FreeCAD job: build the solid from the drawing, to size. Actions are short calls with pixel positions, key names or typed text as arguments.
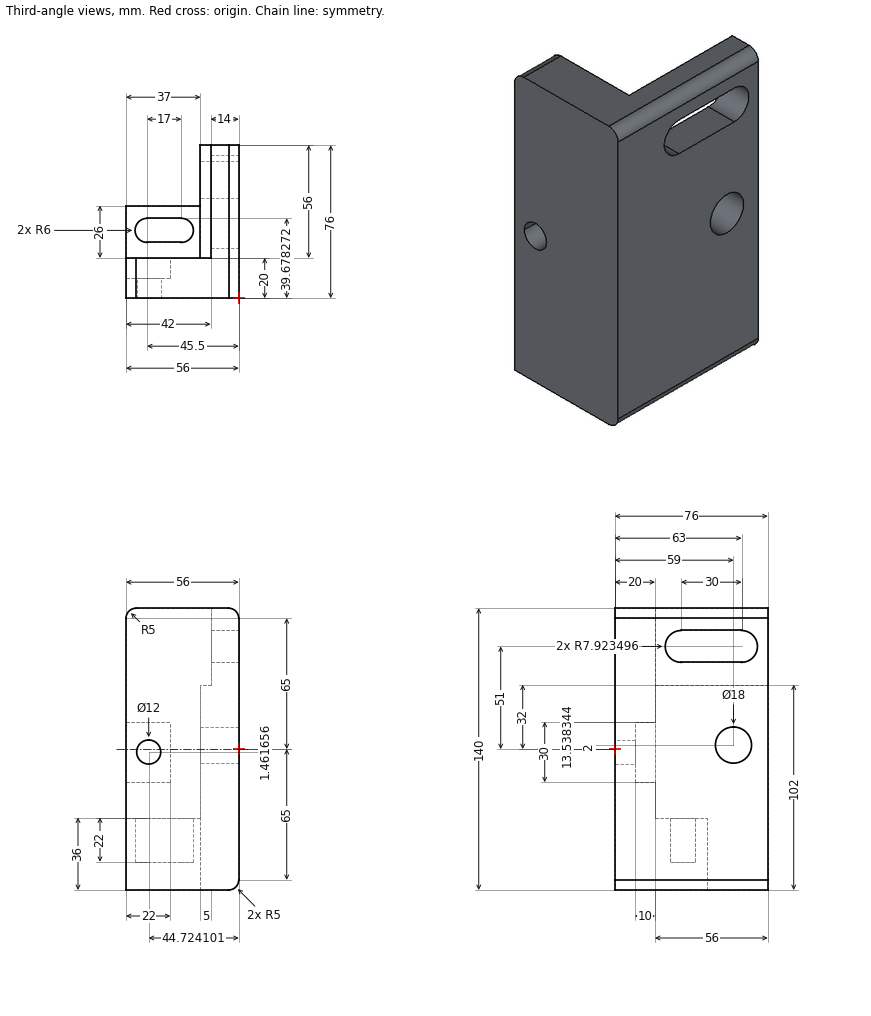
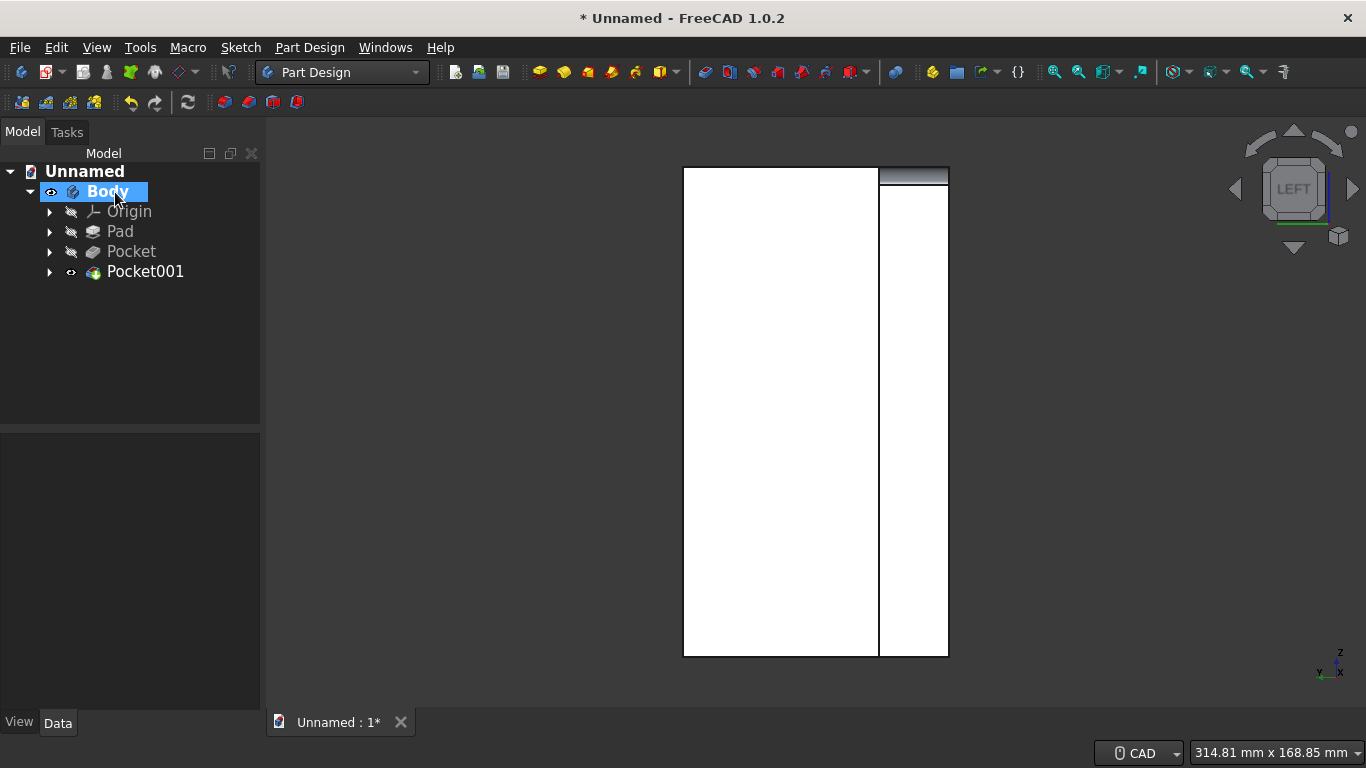
click(781, 271)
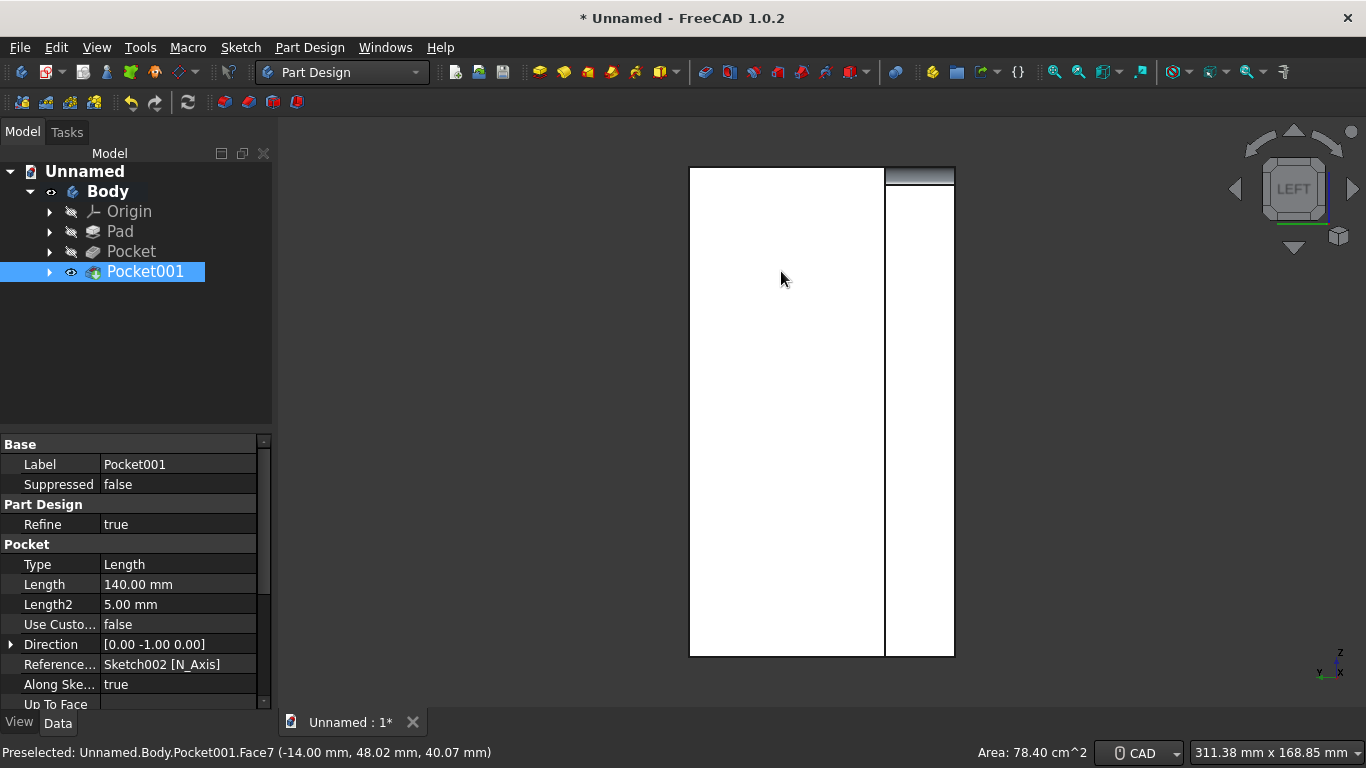
click(46, 72)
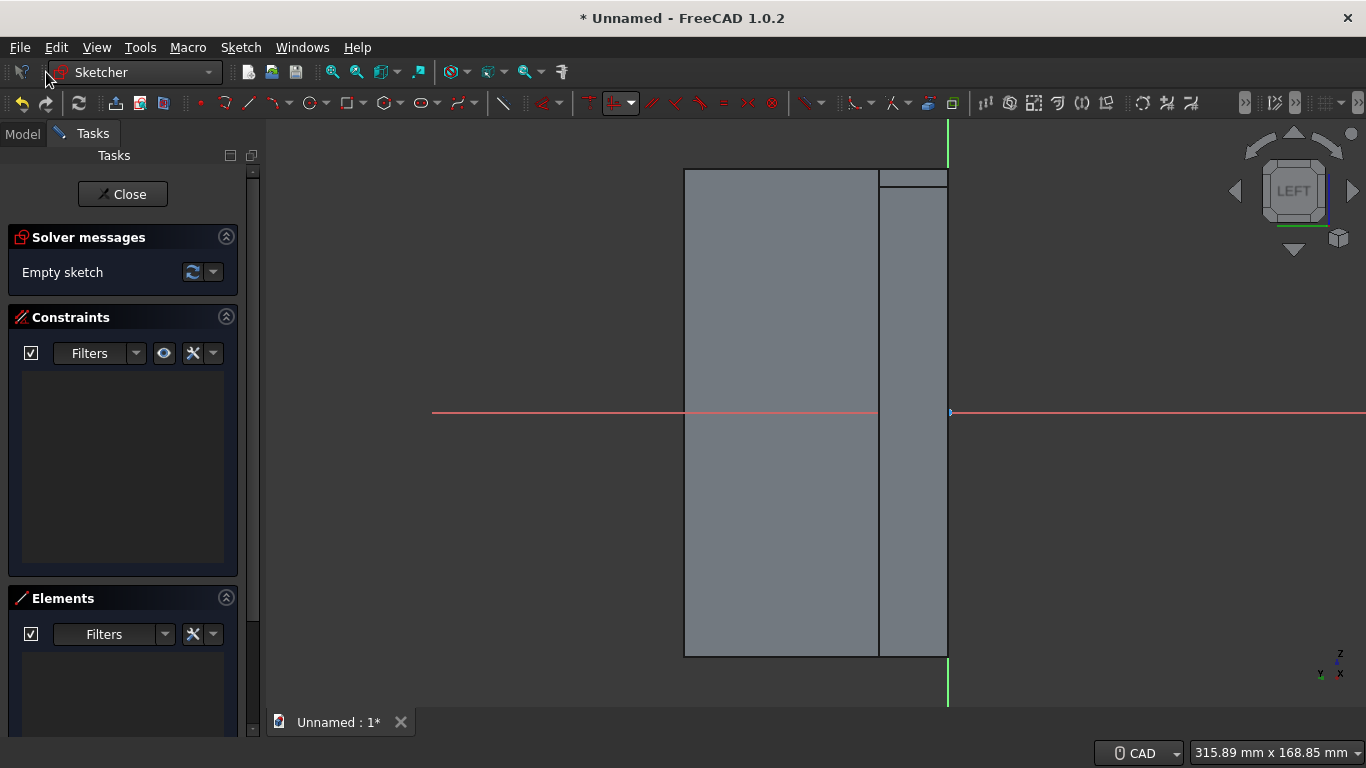
scroll(438, 147, down, 1)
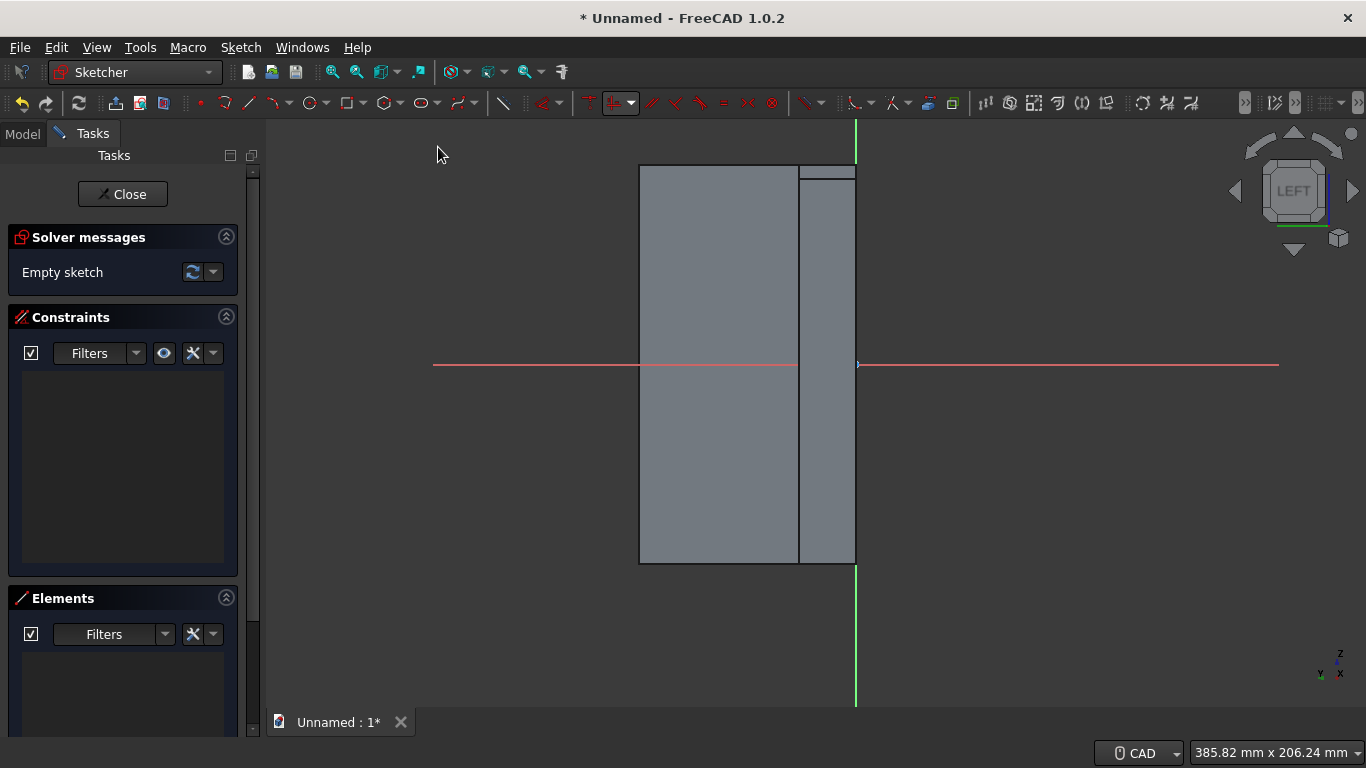
click(348, 104)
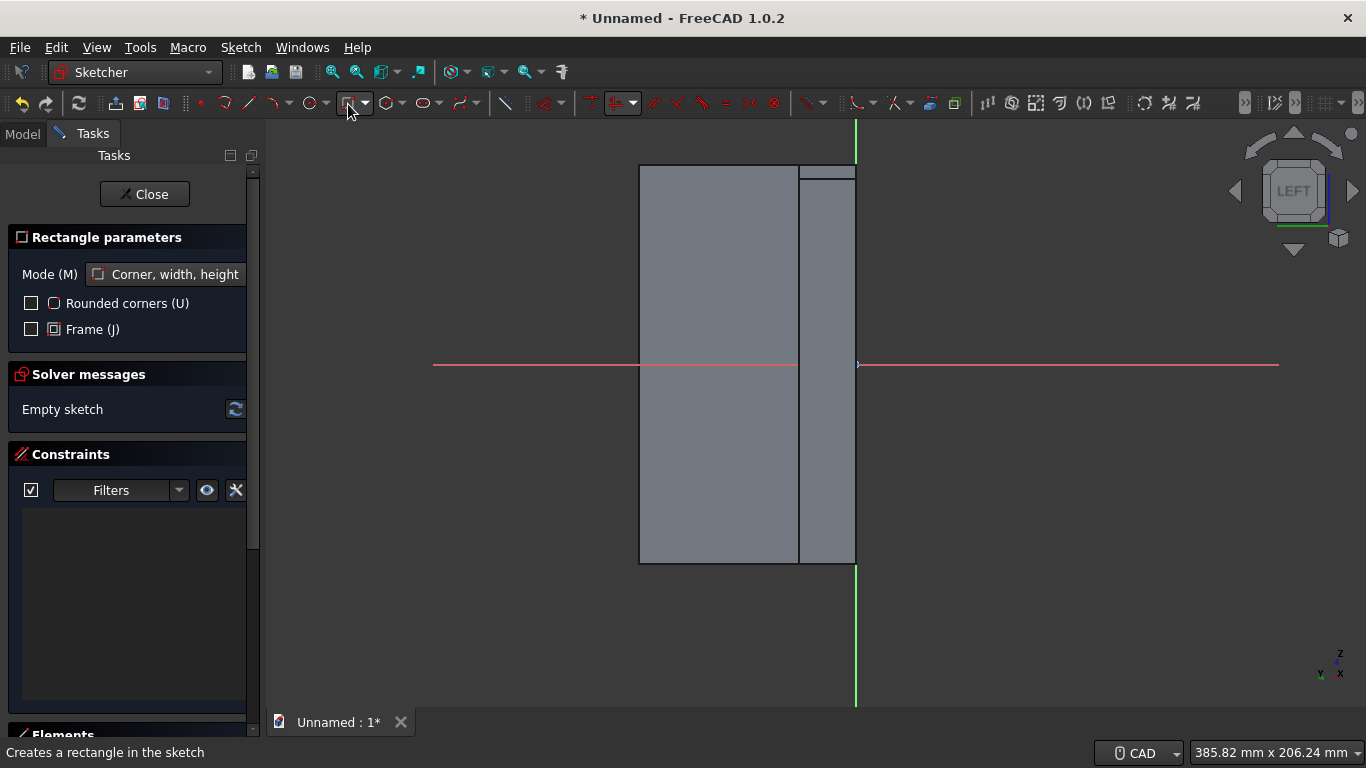
click(639, 274)
click(799, 564)
key(Escape)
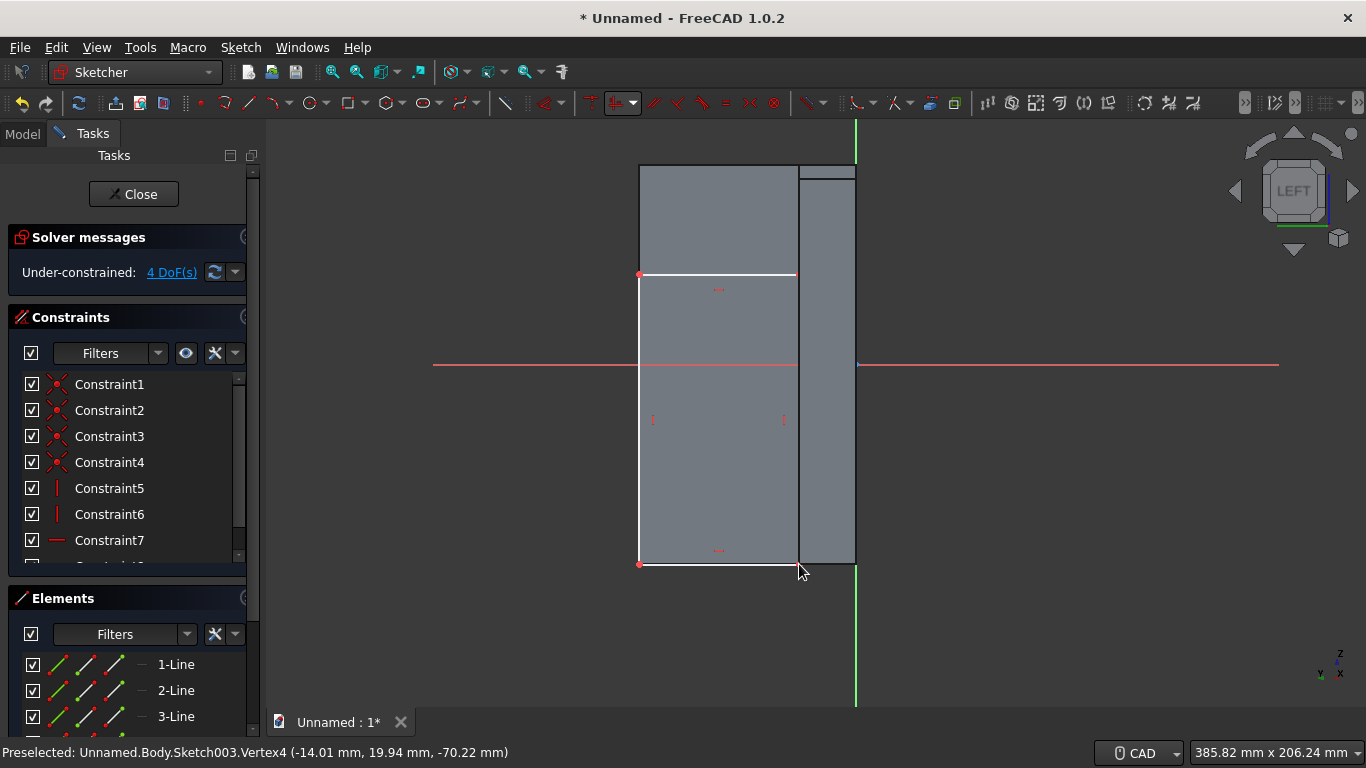
click(544, 104)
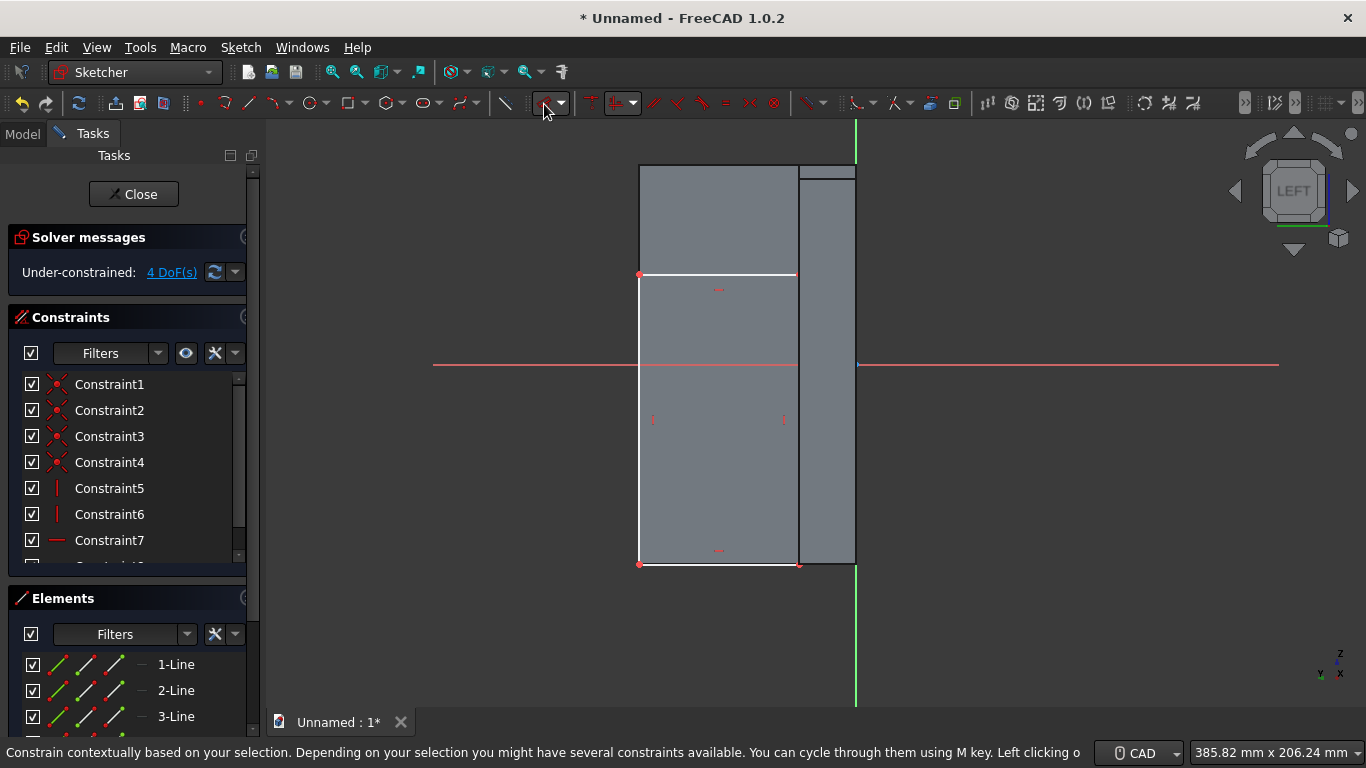
click(687, 565)
click(719, 599)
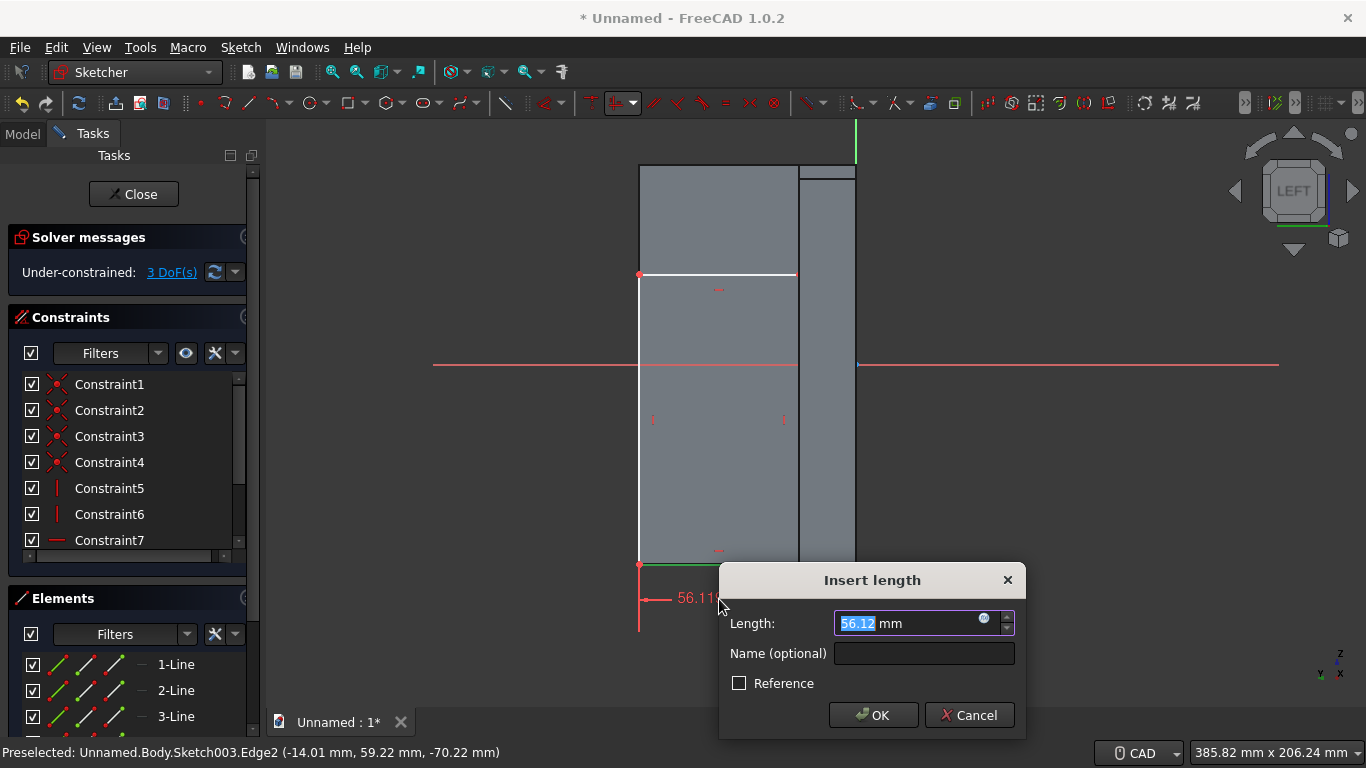
text(56)
key(Return)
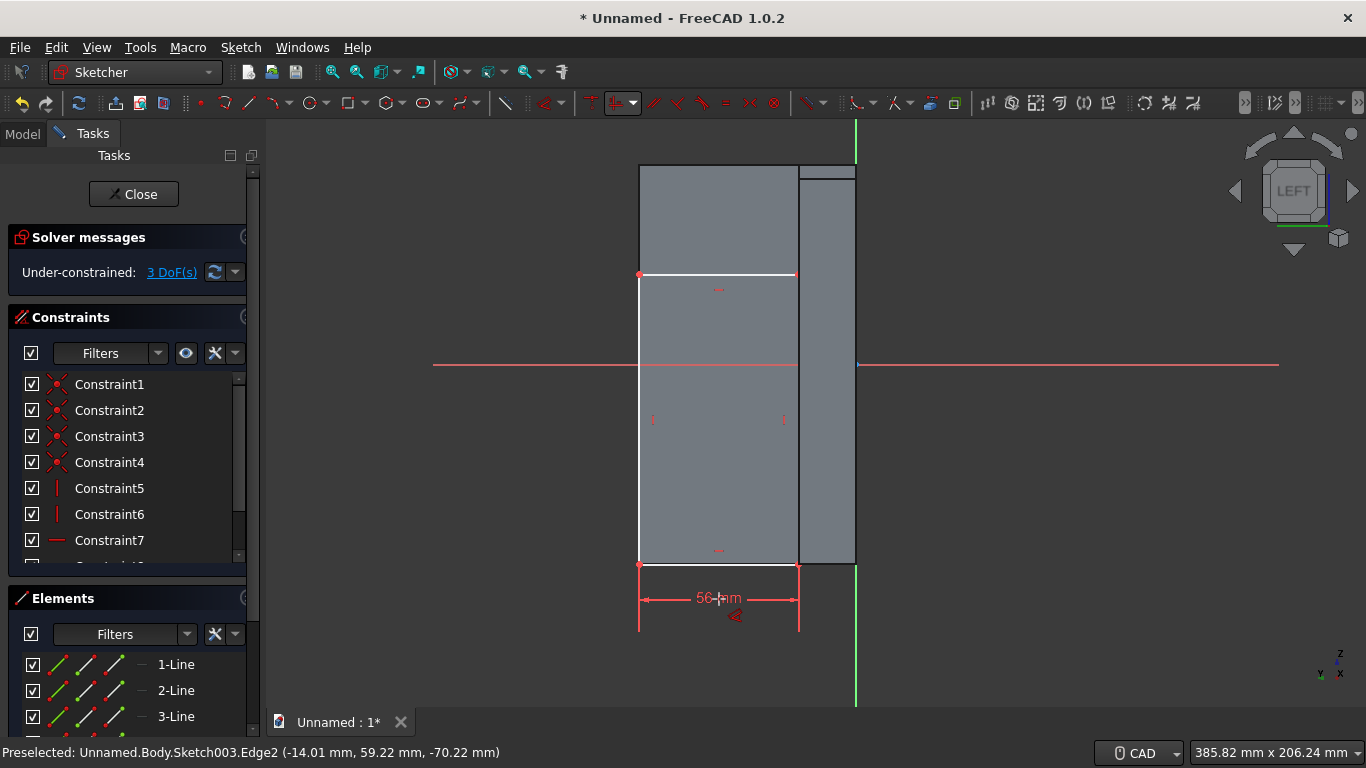
click(639, 362)
click(605, 420)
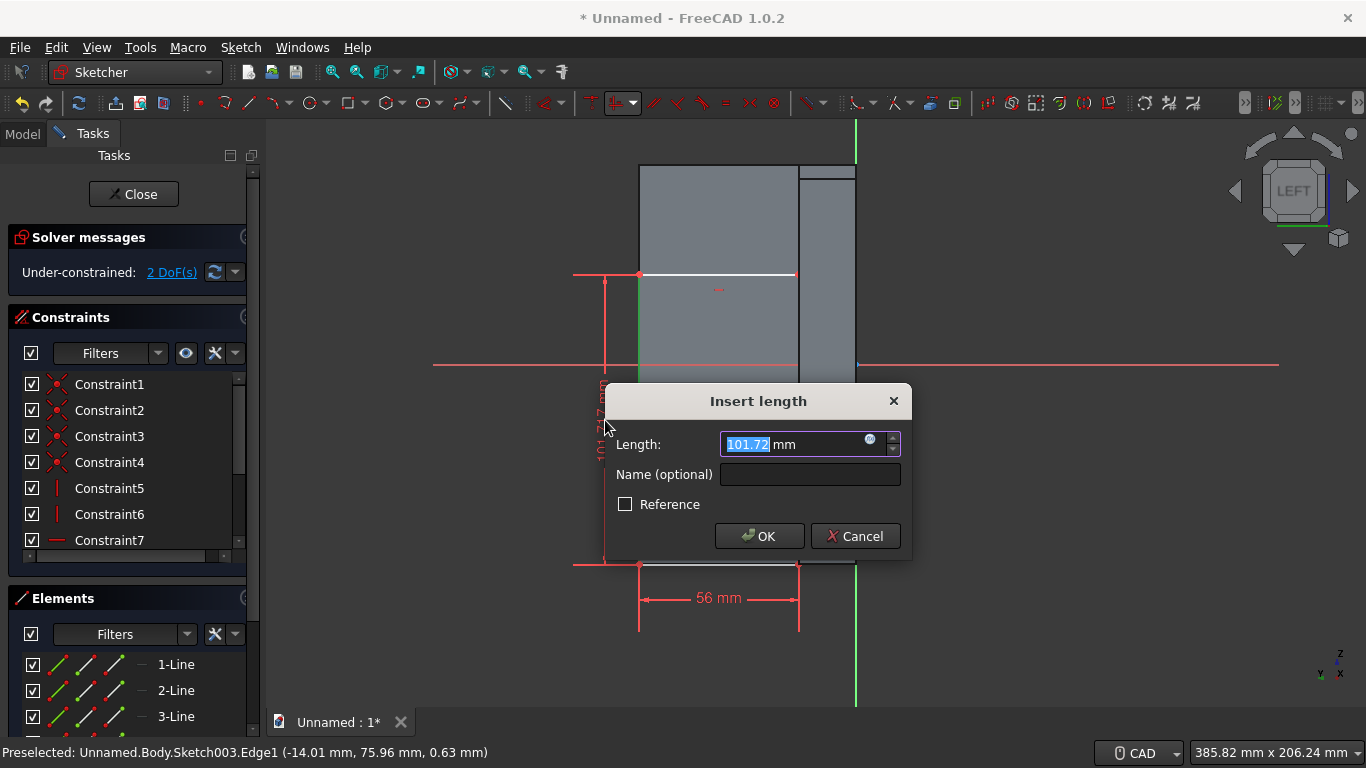
text(102)
key(Return)